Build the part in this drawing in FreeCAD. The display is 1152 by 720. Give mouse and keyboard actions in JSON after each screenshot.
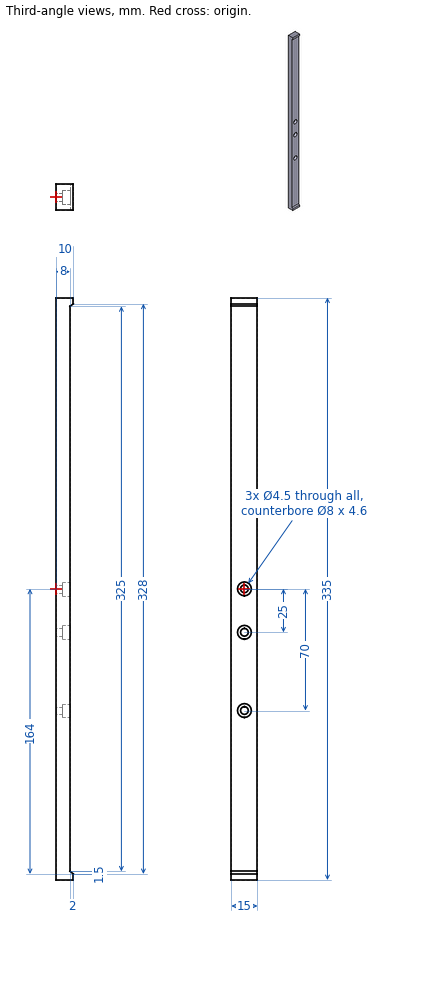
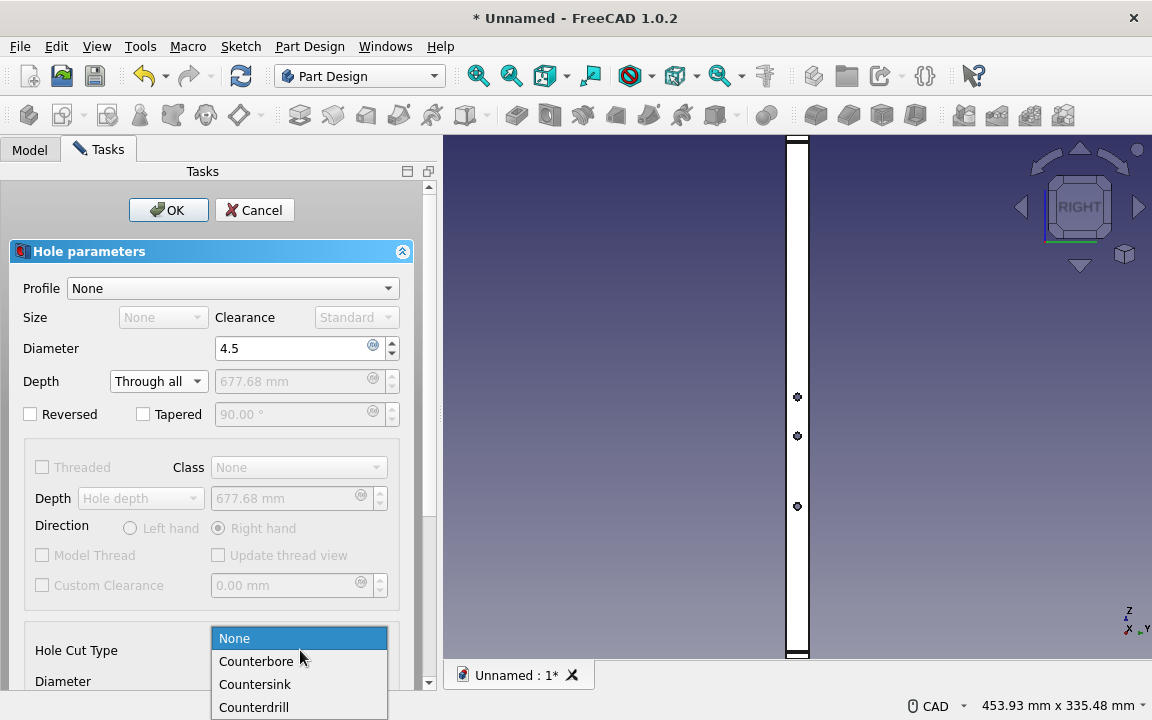
{"action": "left_click", "coordinate": [298, 662]}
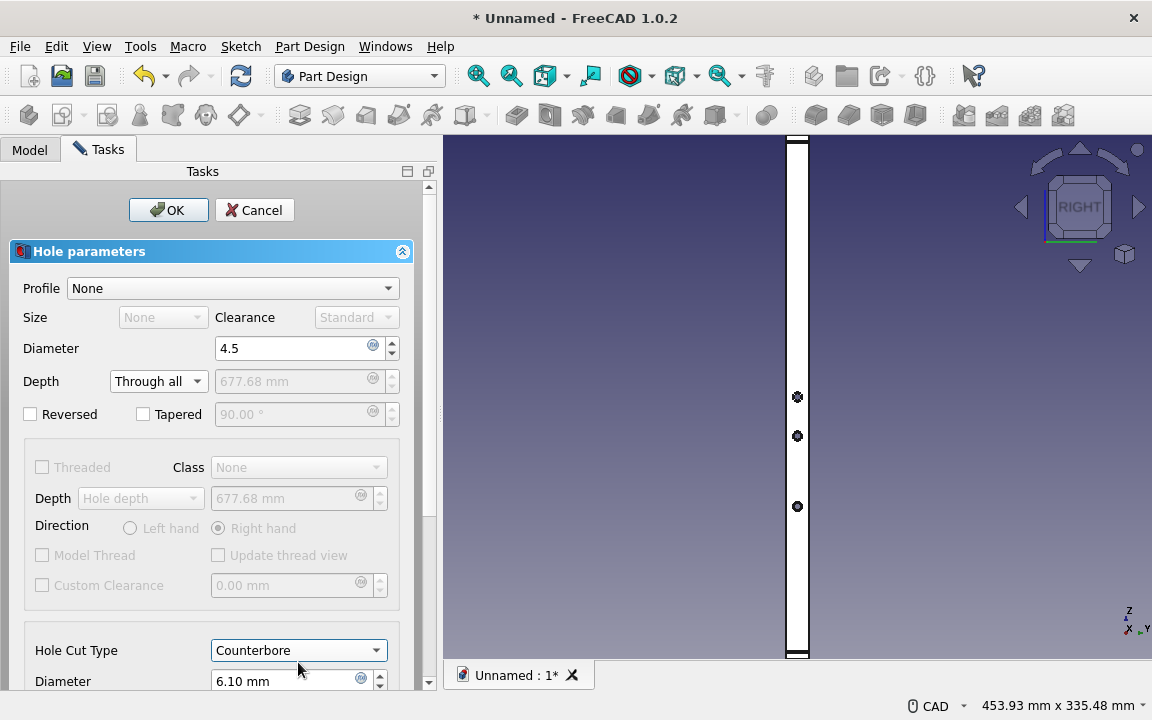
{"action": "scroll", "coordinate": [429, 436], "scroll_direction": "down", "scroll_amount": 2}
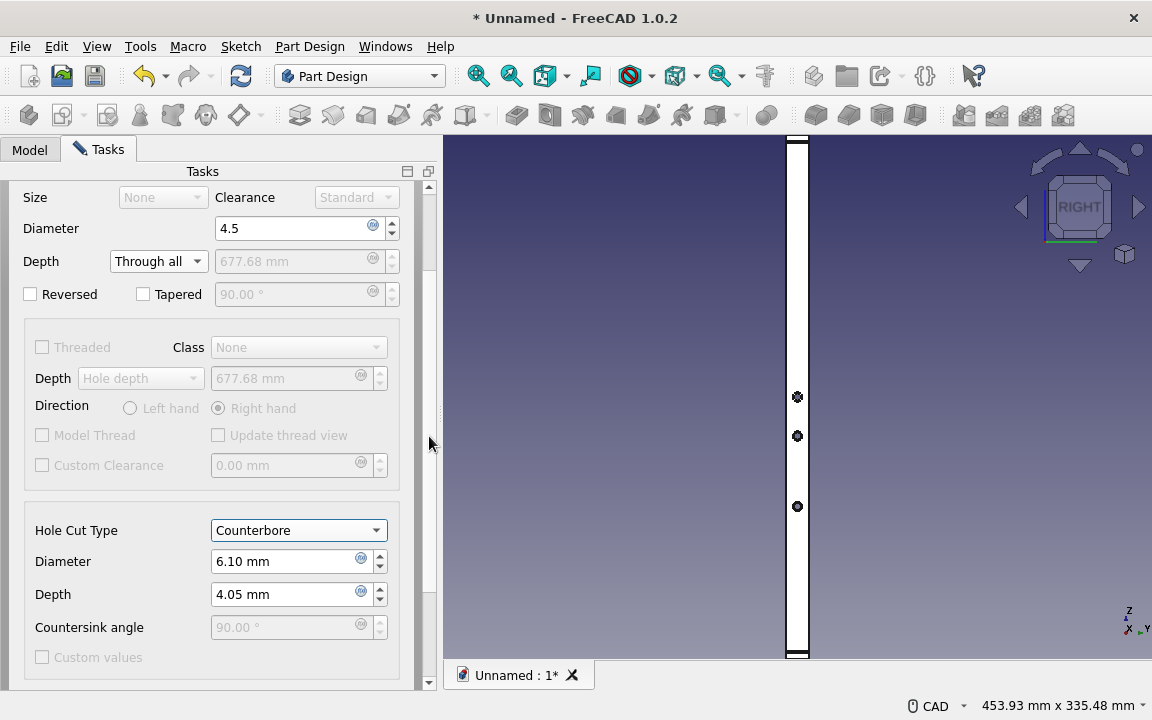
{"action": "triple_click", "coordinate": [292, 562]}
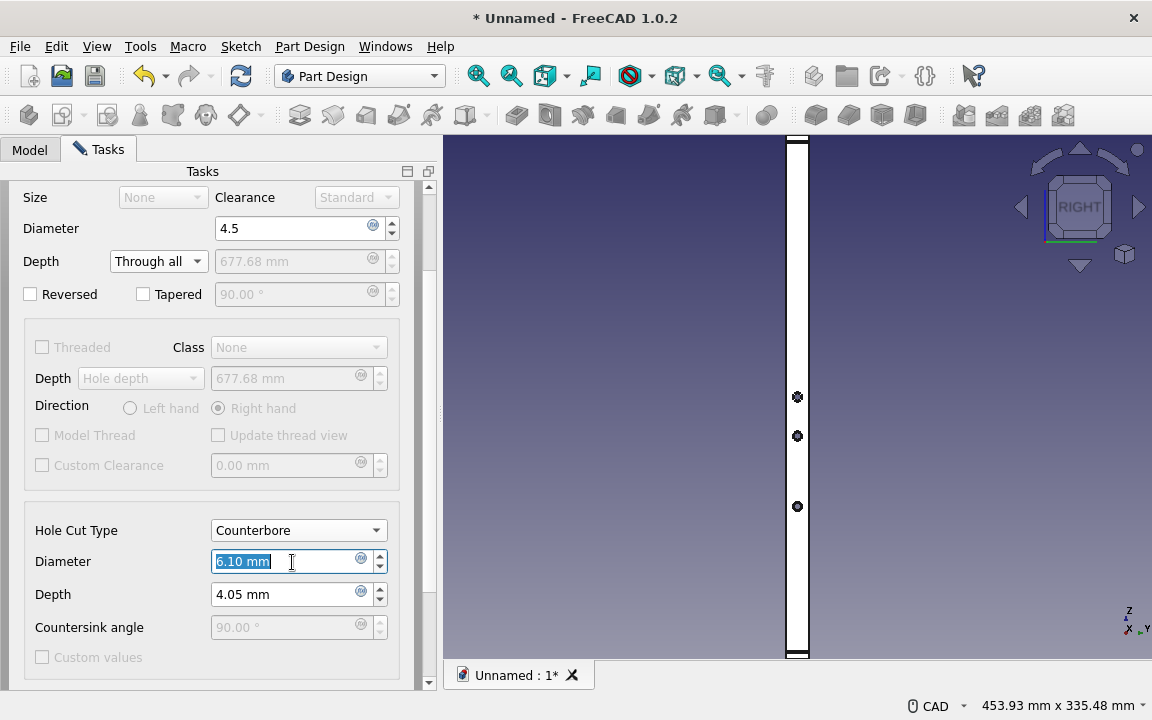
{"action": "type", "text": "8"}
{"action": "key", "text": "Tab"}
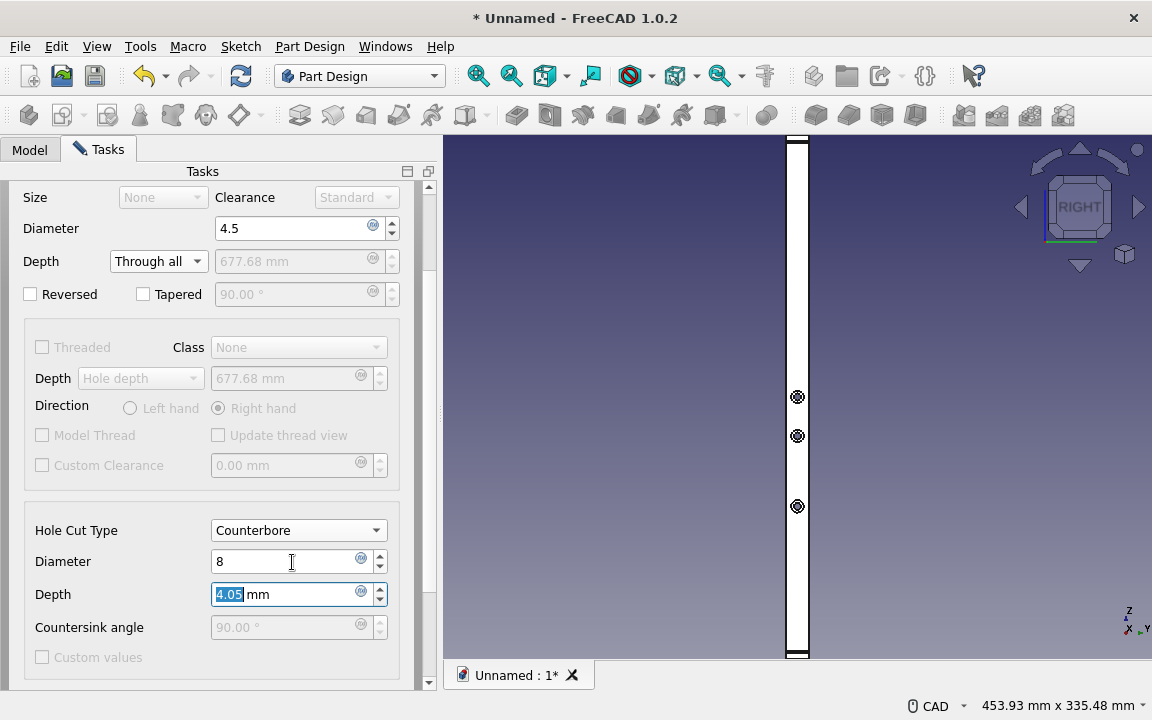
{"action": "type", "text": "4.6"}
{"action": "key", "text": "Tab"}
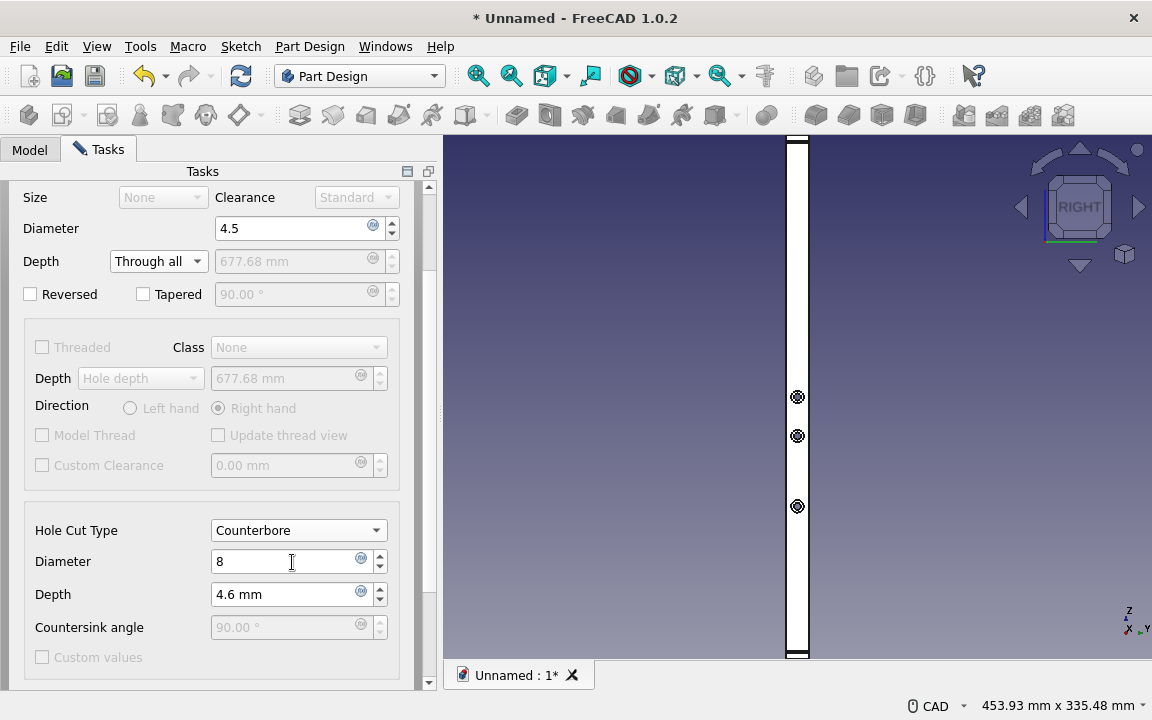
{"action": "scroll", "coordinate": [429, 436], "scroll_direction": "up", "scroll_amount": 3}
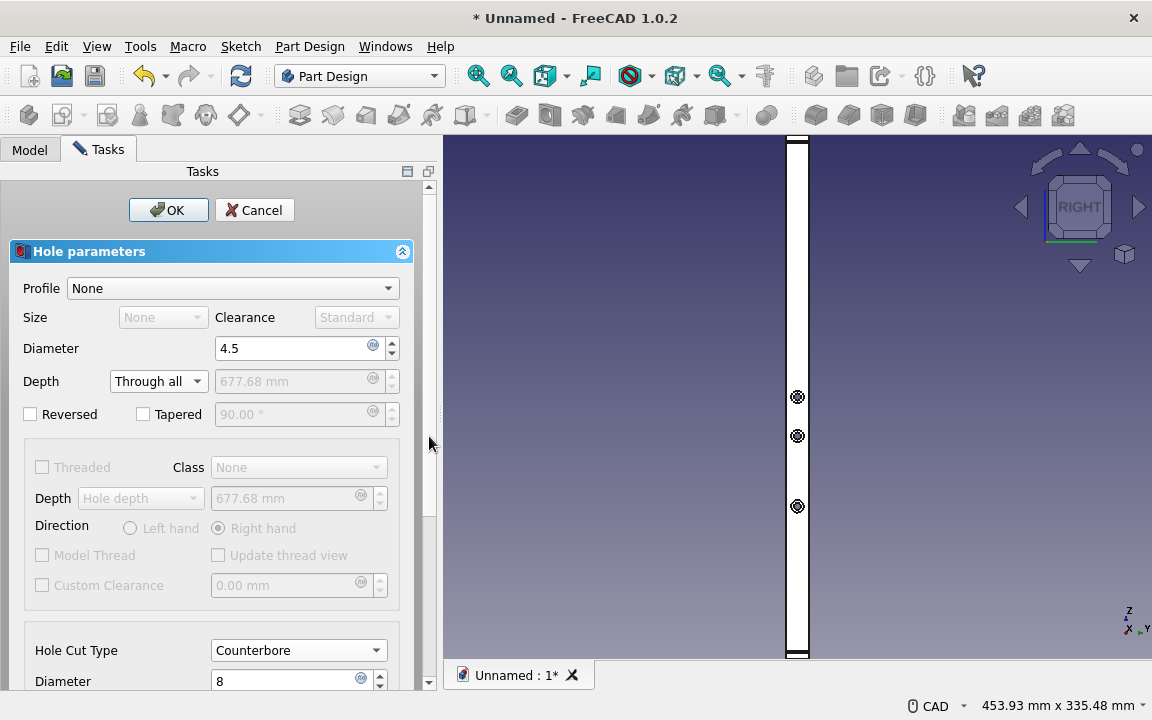
{"action": "left_click", "coordinate": [169, 210]}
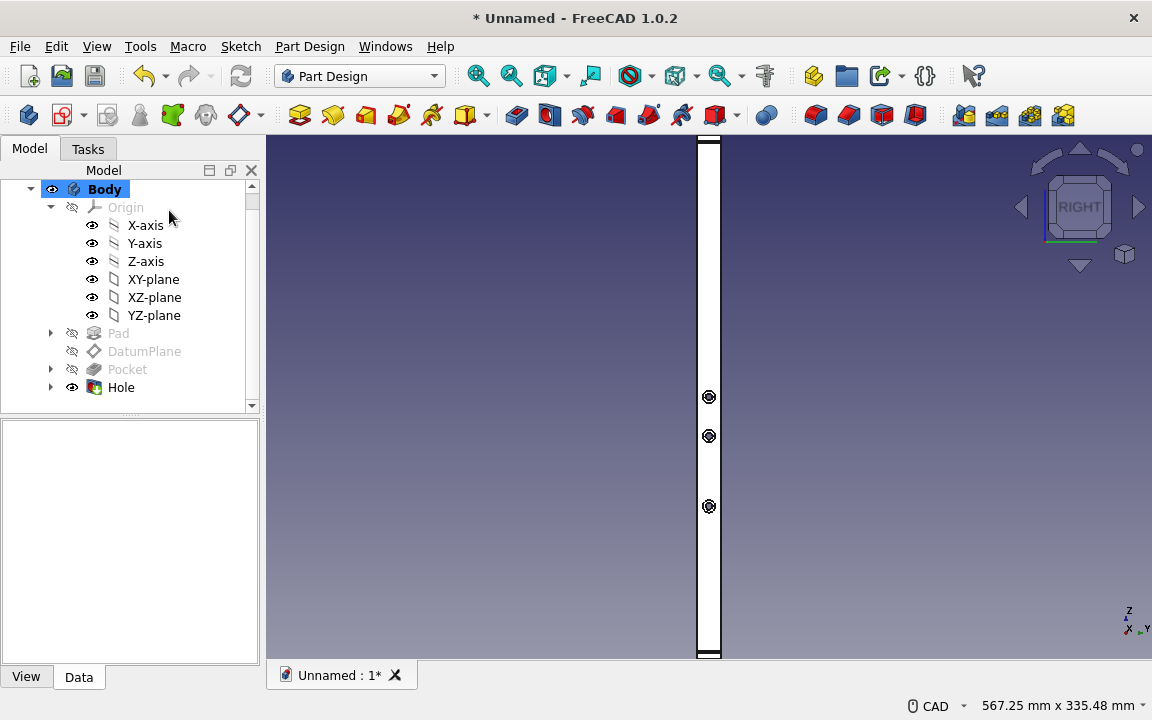
{"action": "key", "text": "0"}